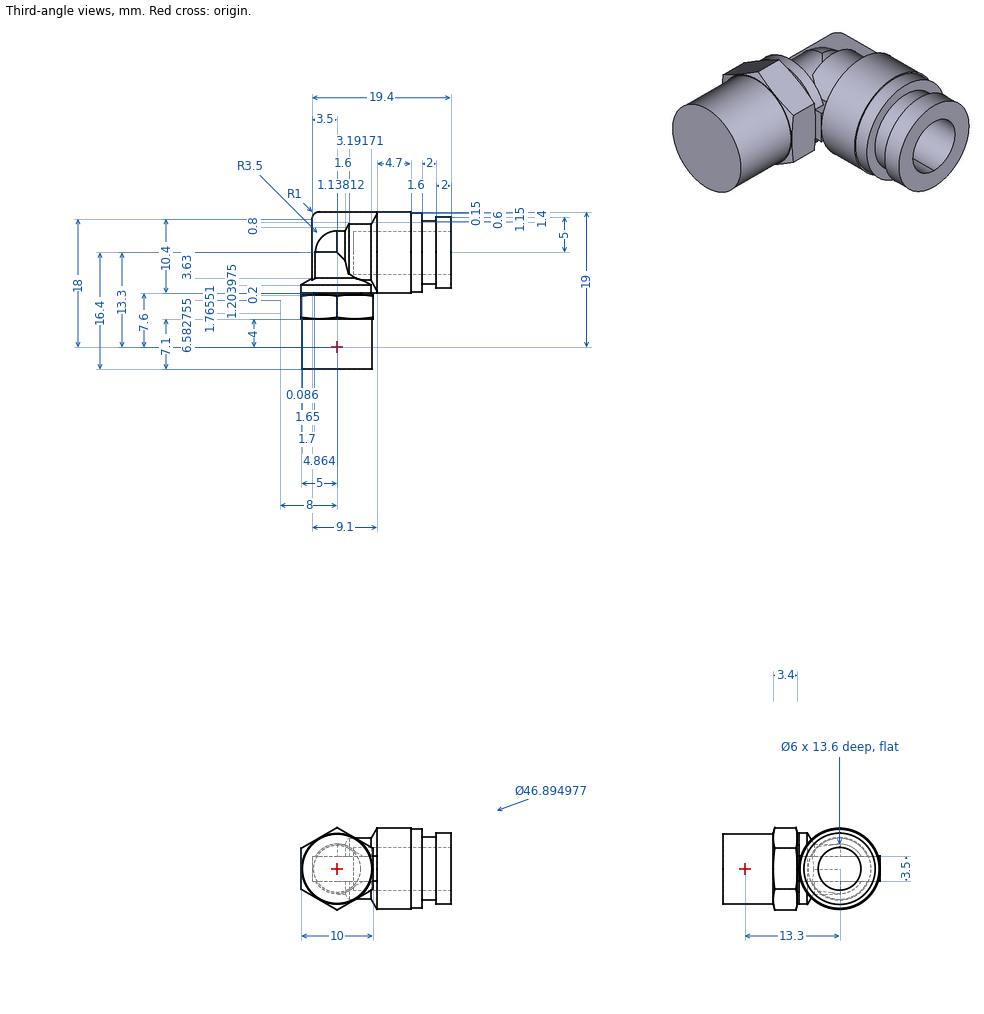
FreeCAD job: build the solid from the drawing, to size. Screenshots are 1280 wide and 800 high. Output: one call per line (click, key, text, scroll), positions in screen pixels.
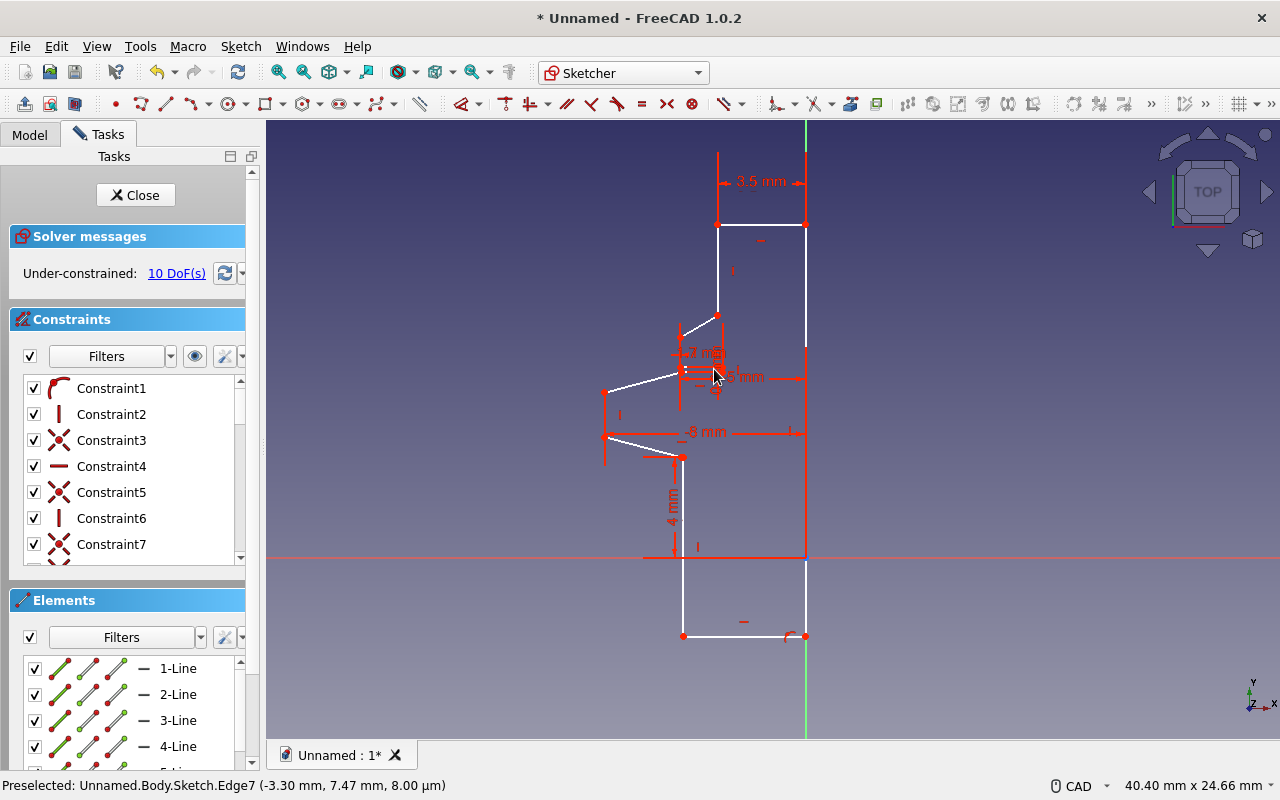
click(683, 511)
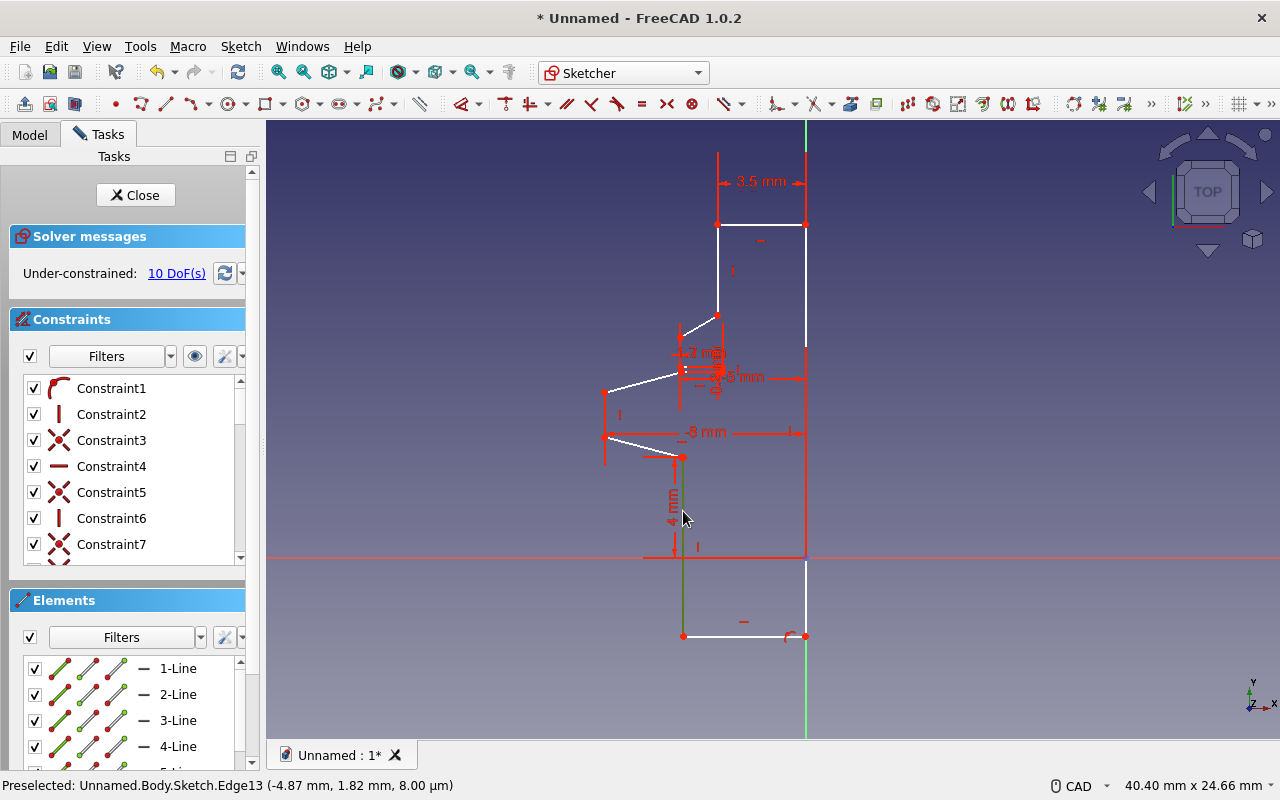
key(i)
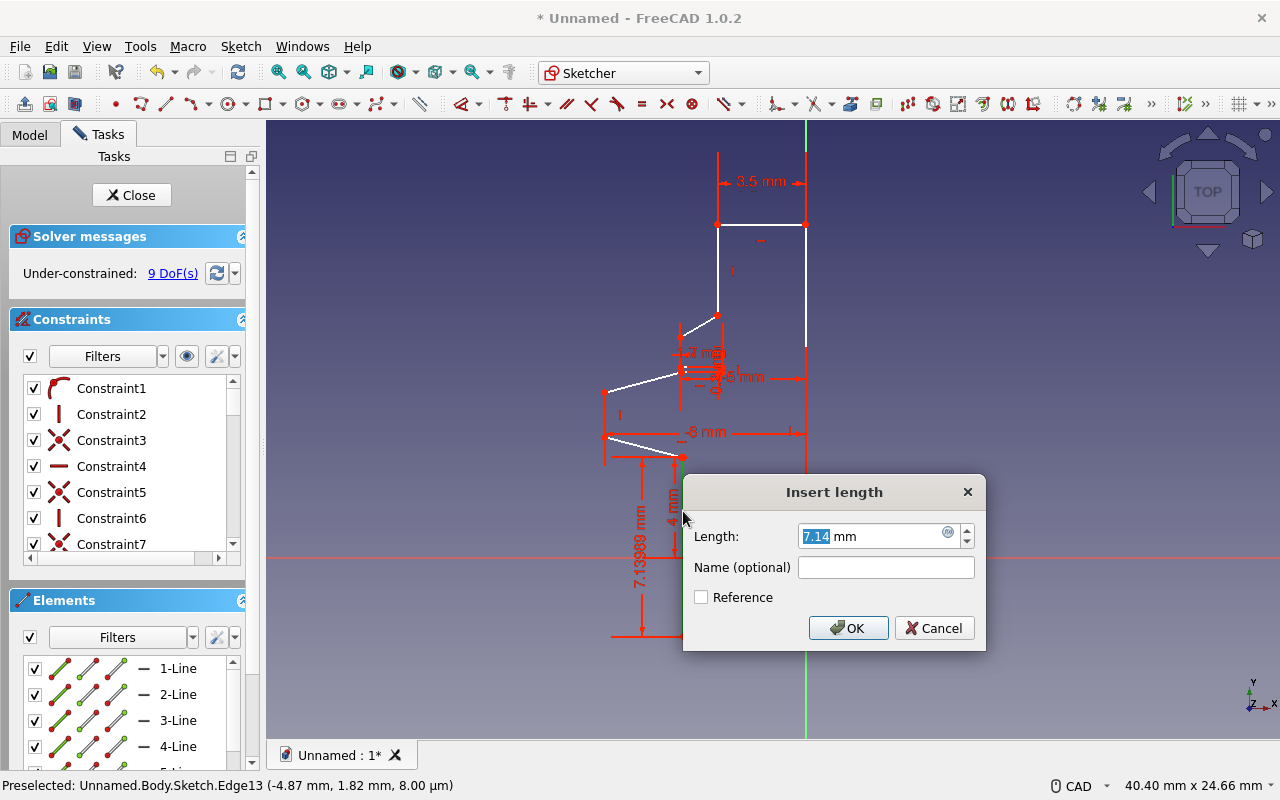
text(7.1)
key(Return)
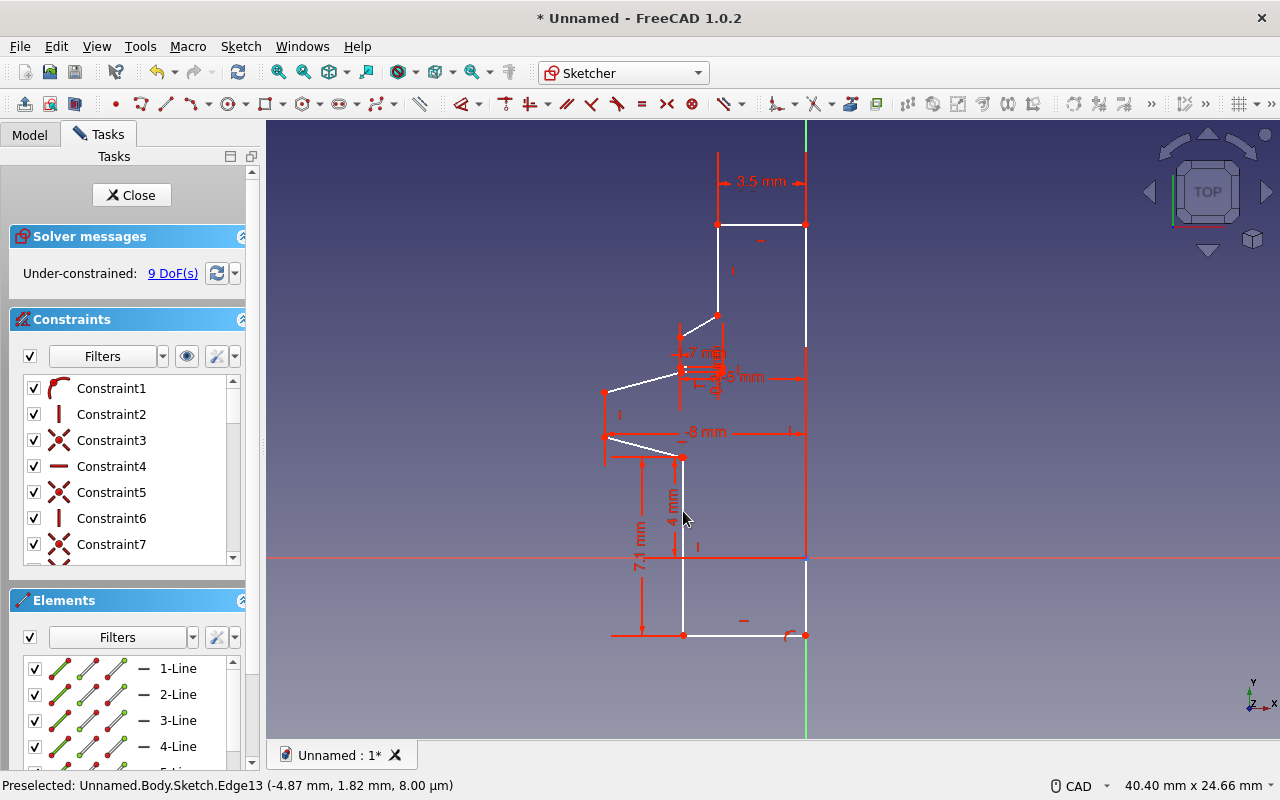
click(806, 512)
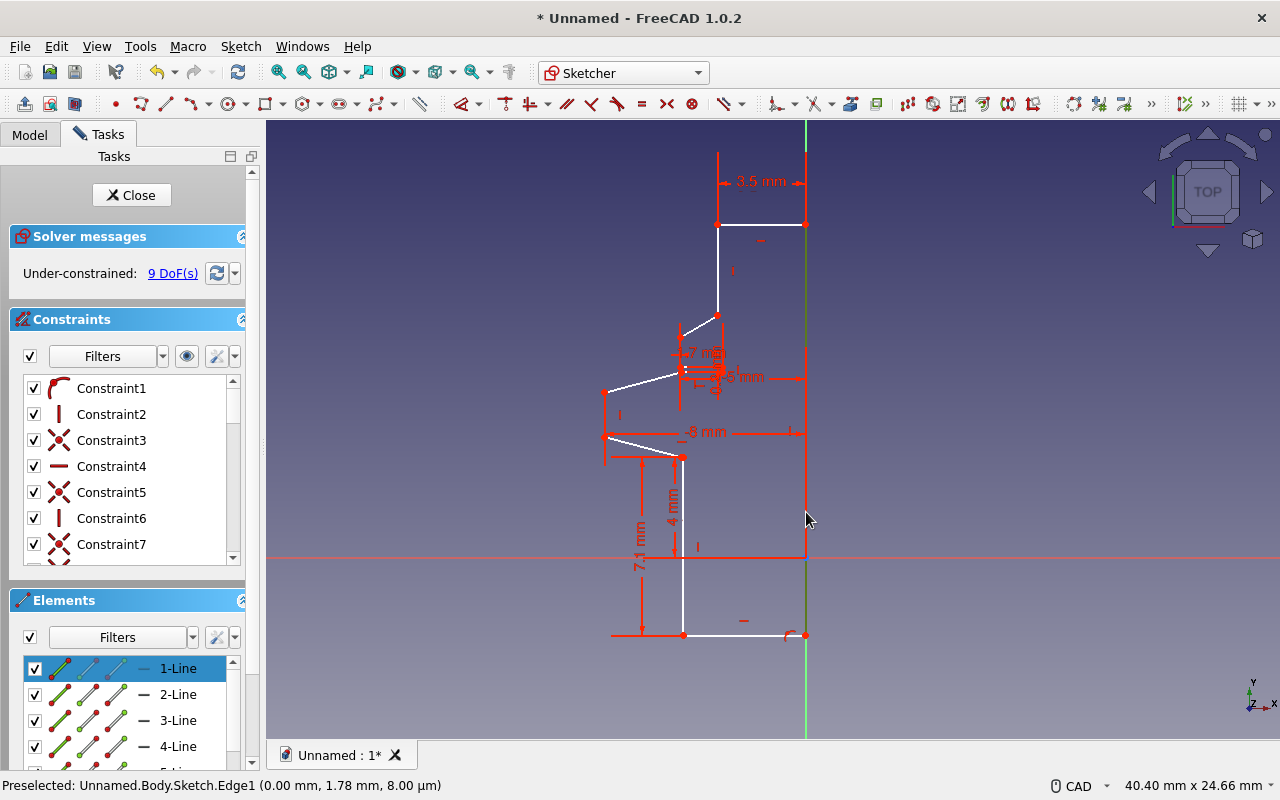
key(i)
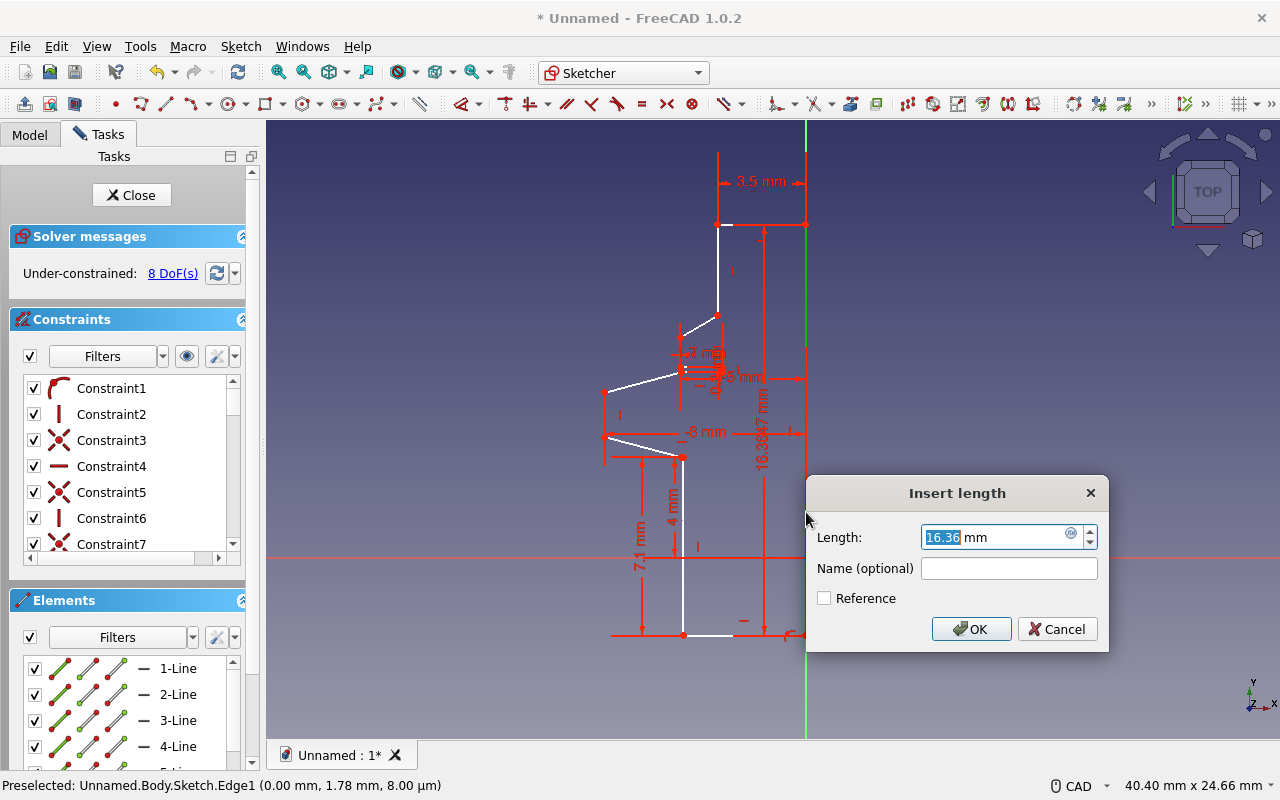
text(16.4)
key(Return)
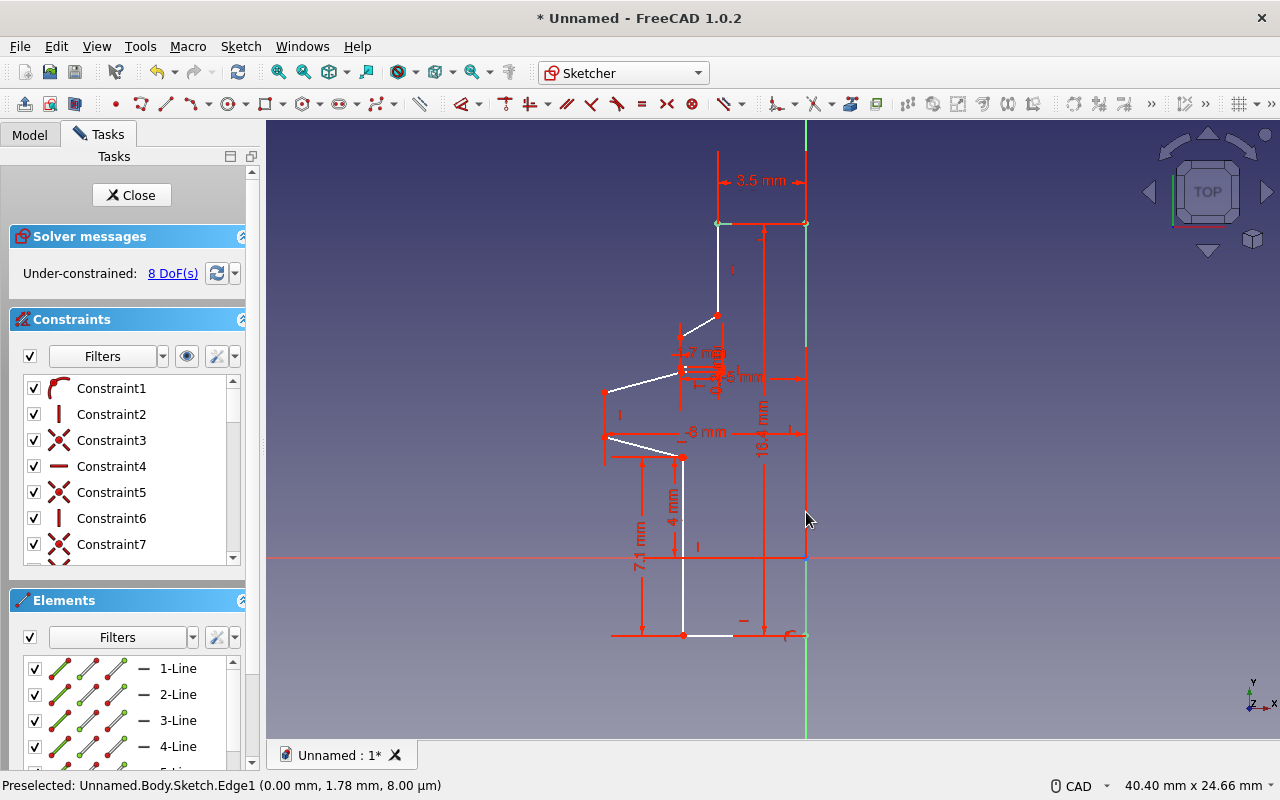
click(718, 251)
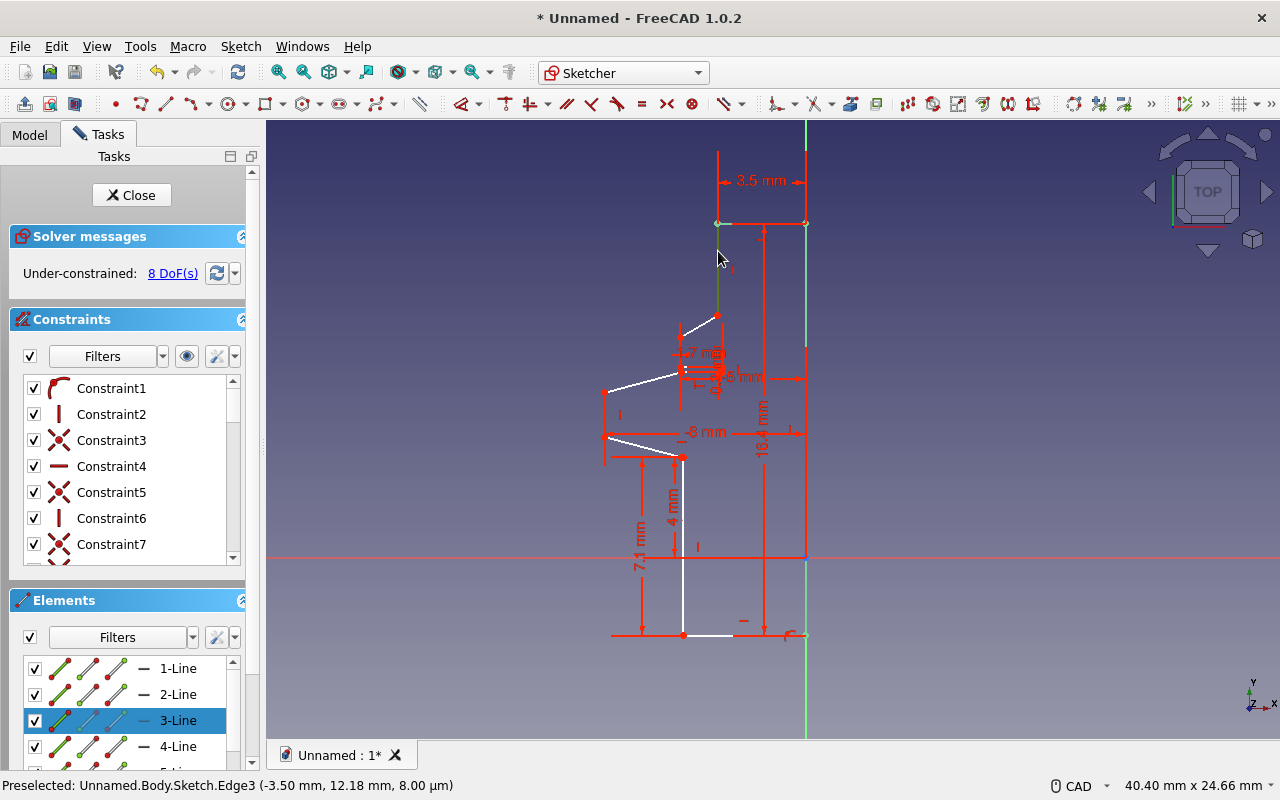
key(i)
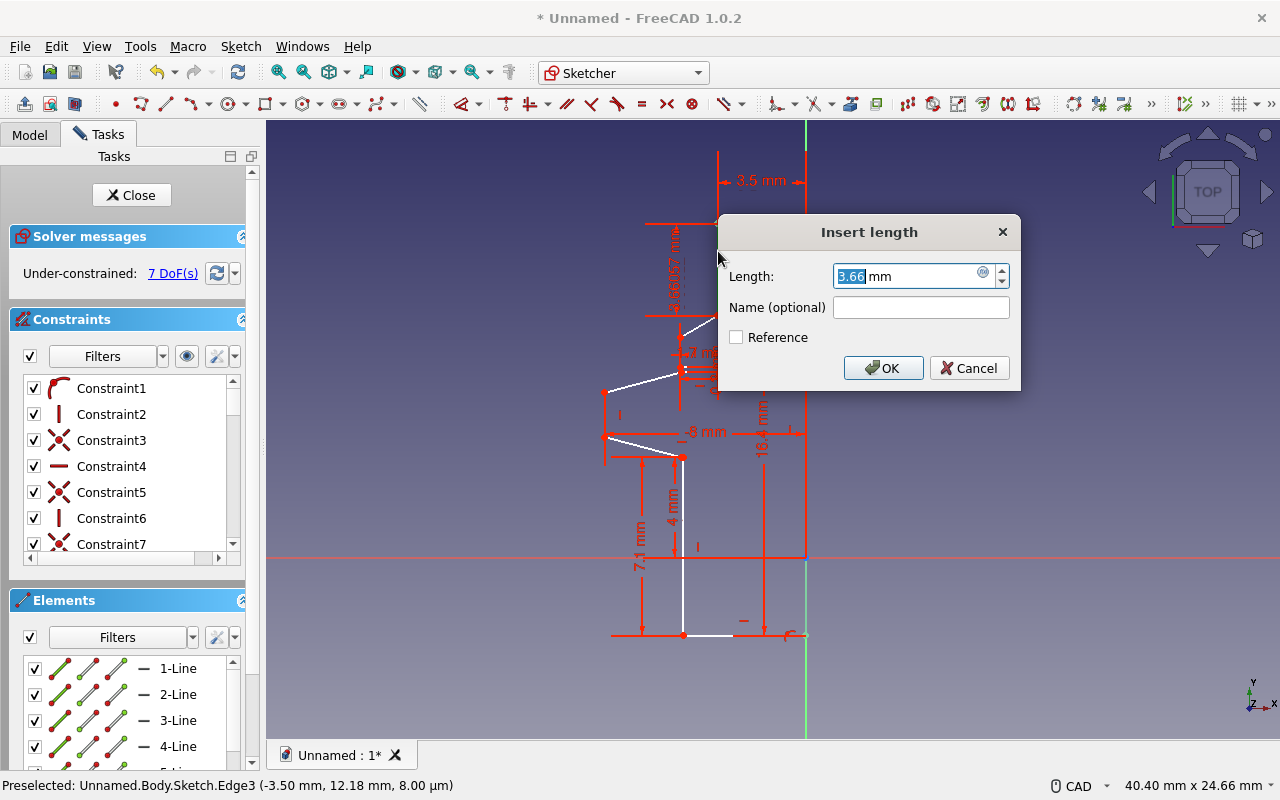
text(3.63)
key(Return)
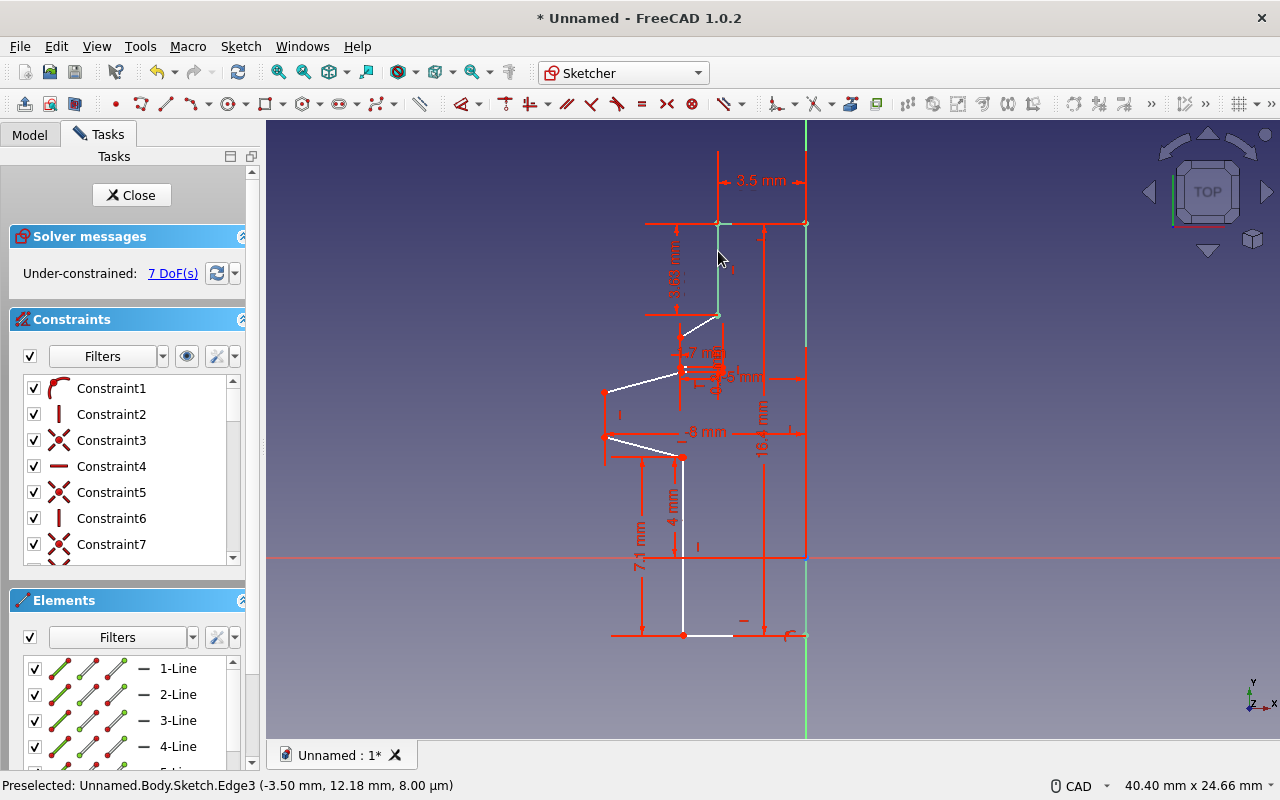
scroll(710, 372, up, 6)